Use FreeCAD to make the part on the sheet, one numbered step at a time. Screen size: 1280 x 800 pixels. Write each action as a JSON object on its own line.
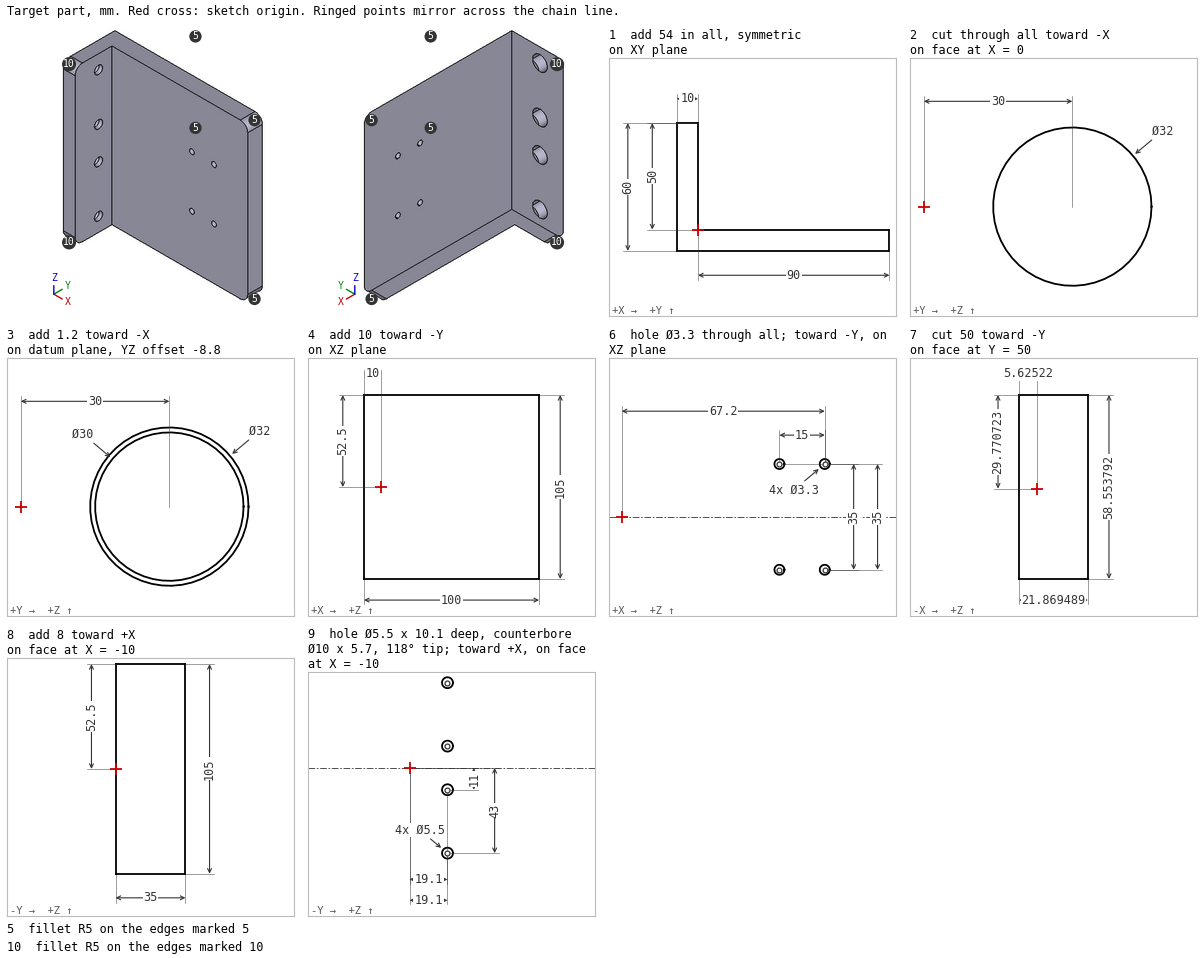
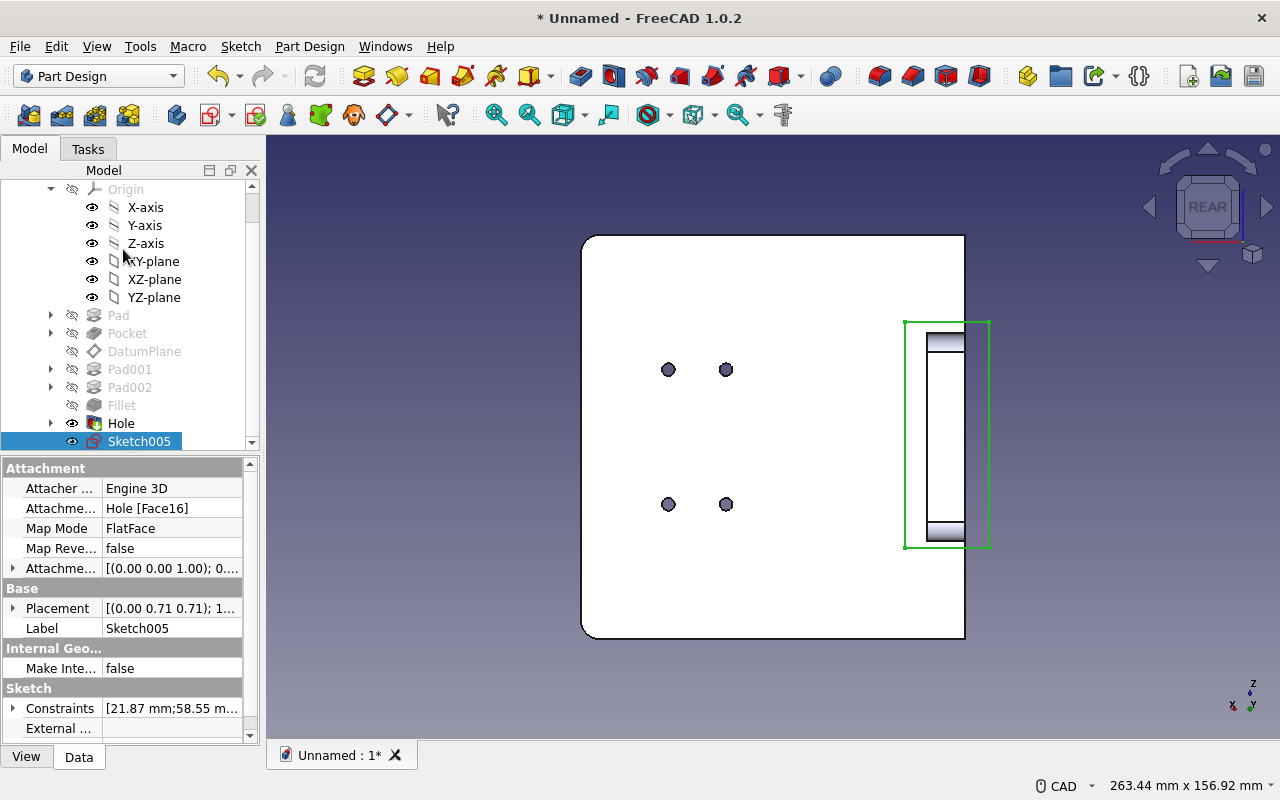
{"action": "left_click", "coordinate": [581, 76]}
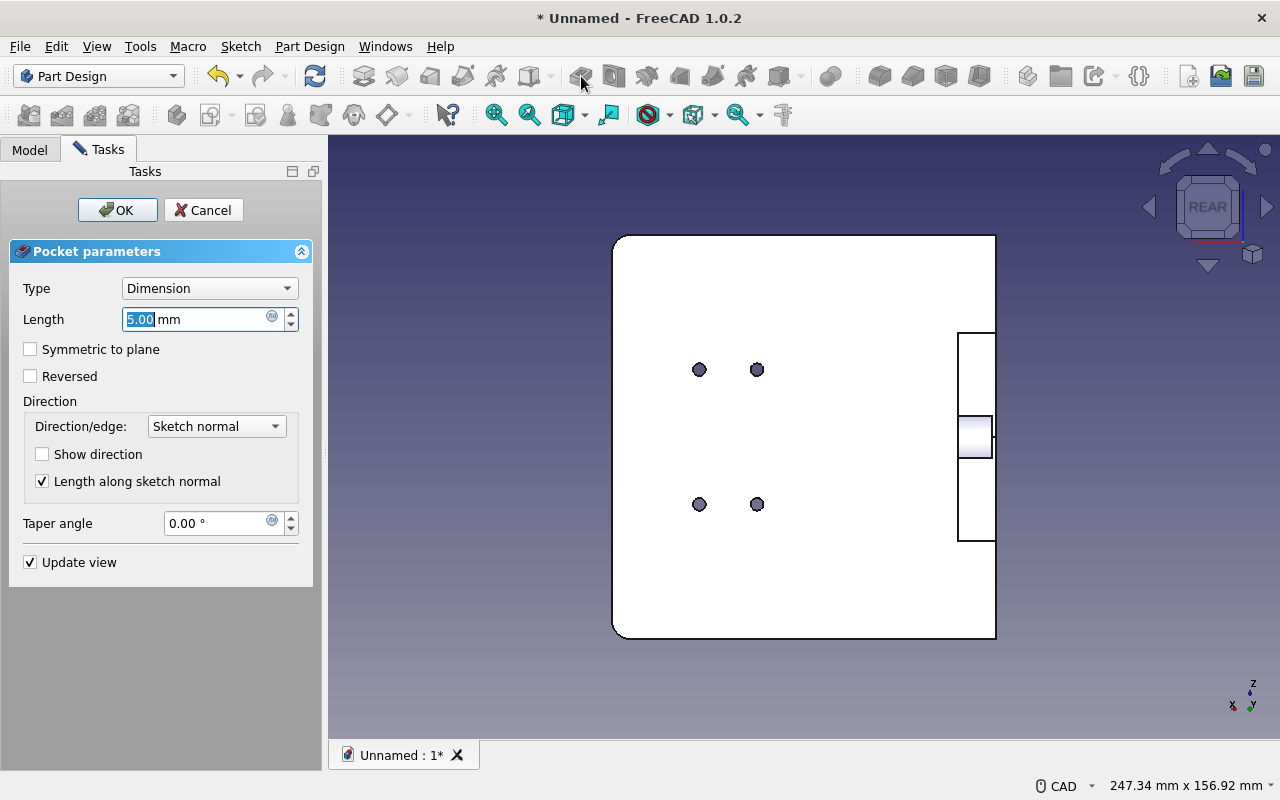
{"action": "type", "text": "50"}
{"action": "key", "text": "Tab"}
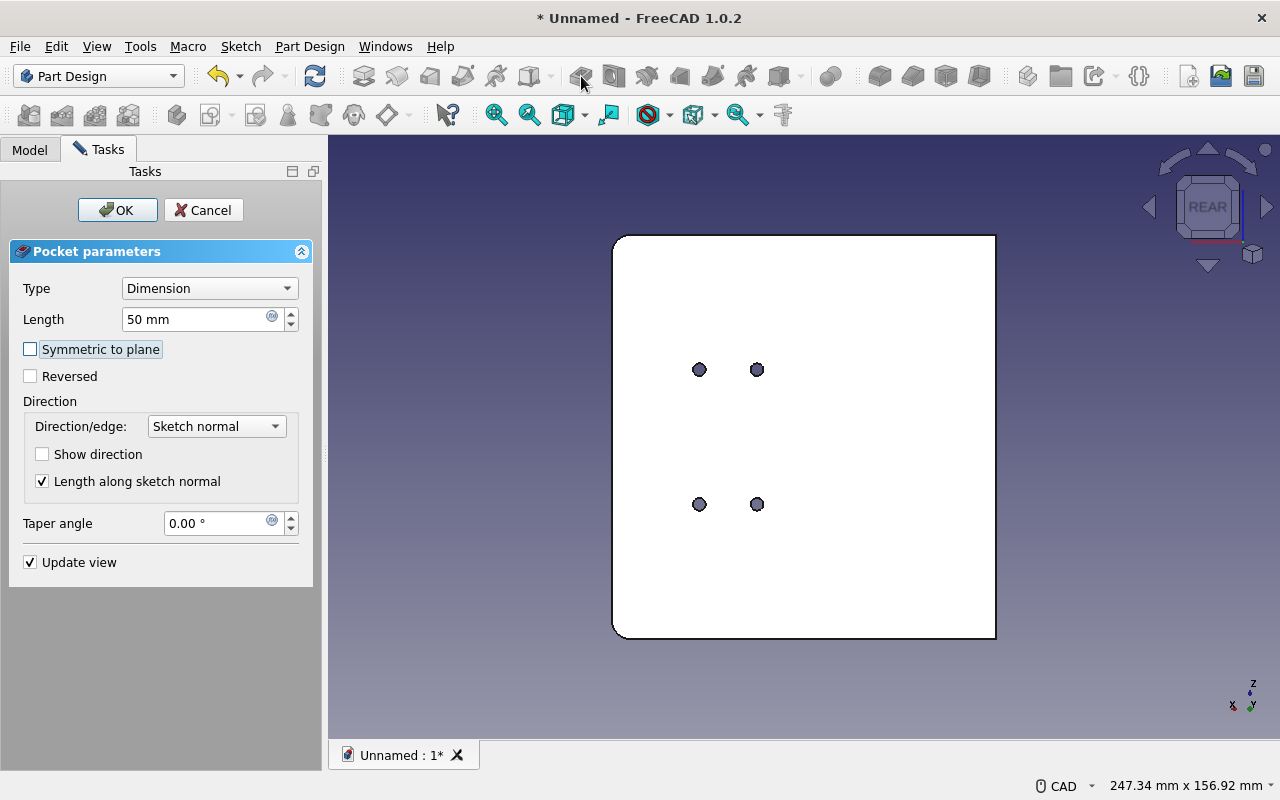
{"action": "left_click", "coordinate": [118, 210]}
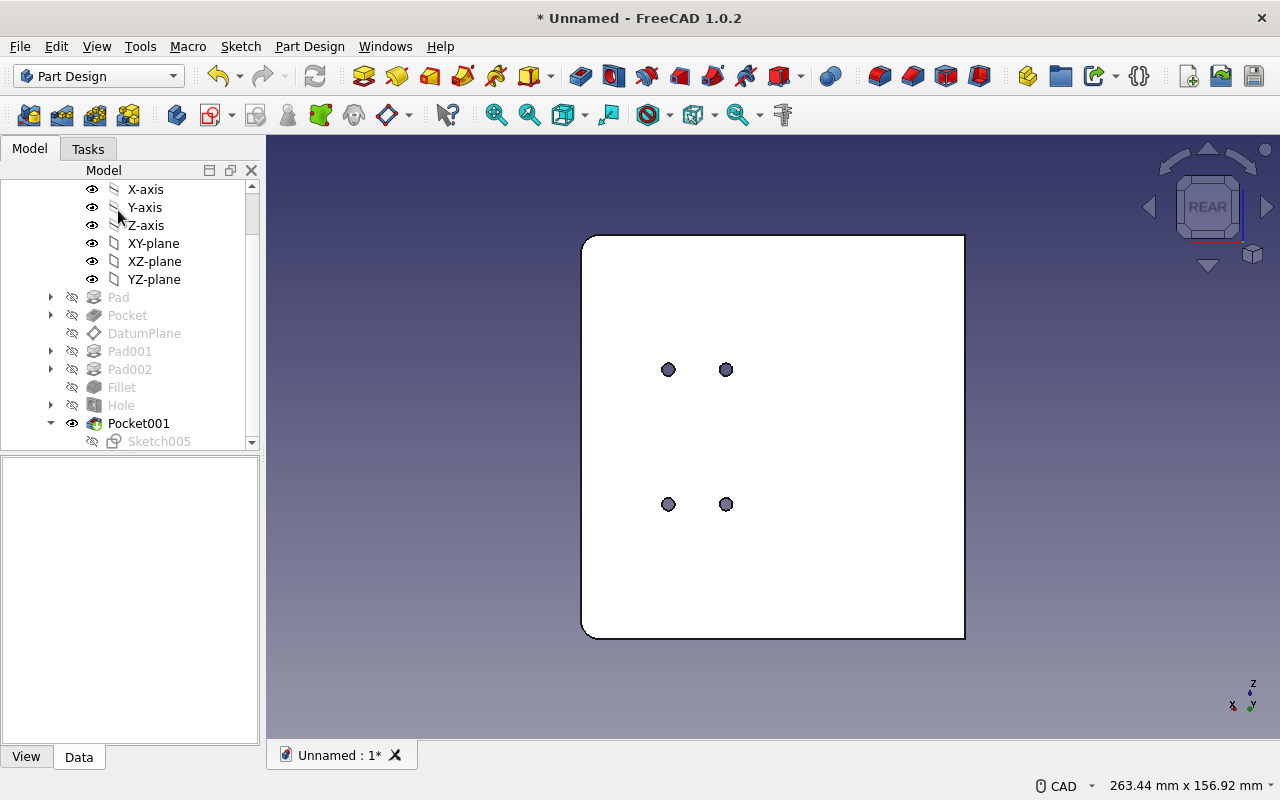
{"action": "key", "text": "6"}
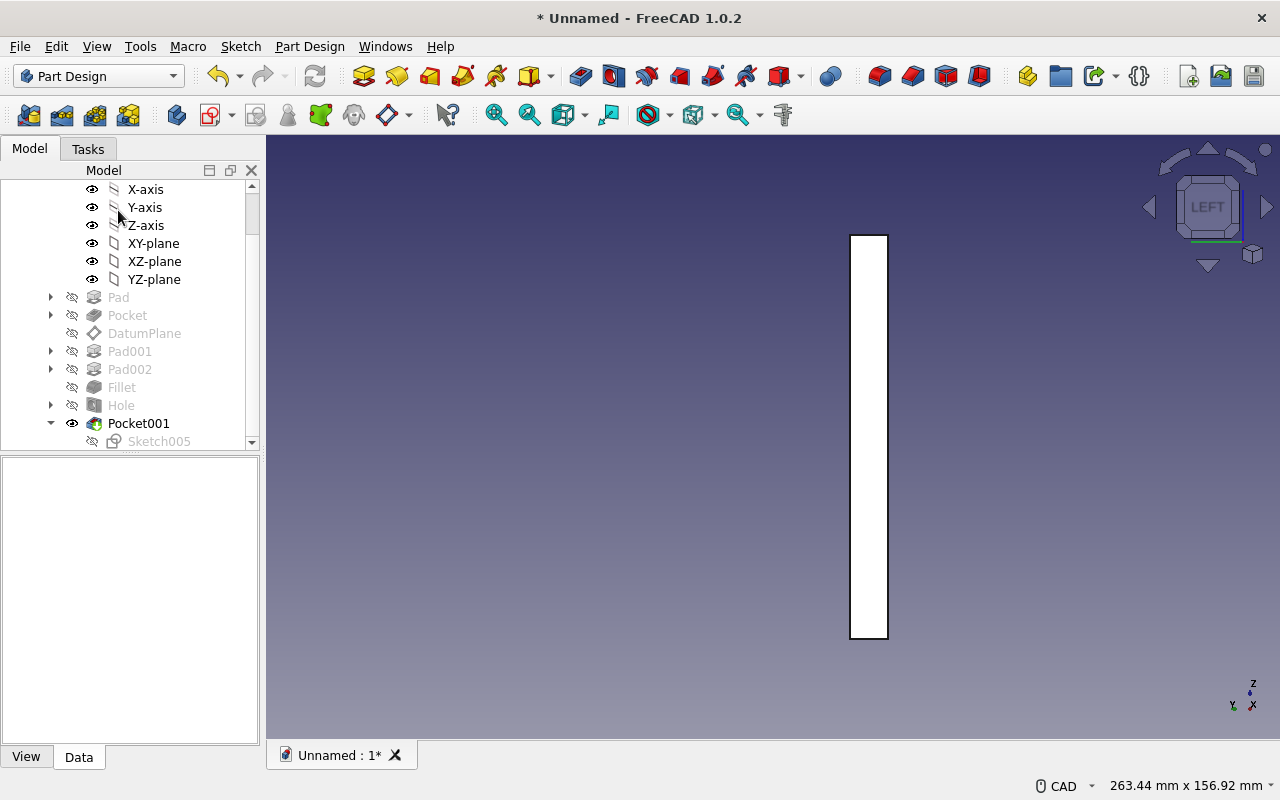
{"action": "left_click", "coordinate": [869, 436]}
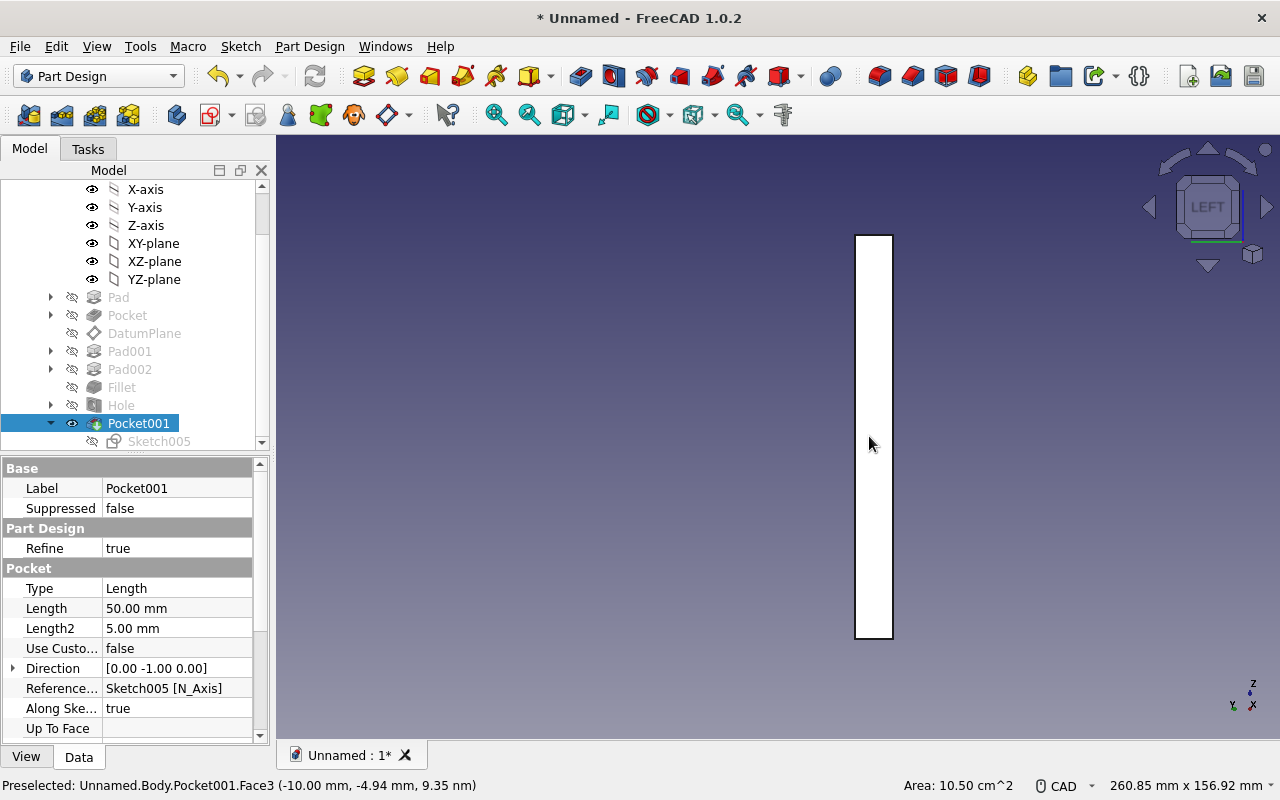
{"action": "left_click", "coordinate": [210, 116]}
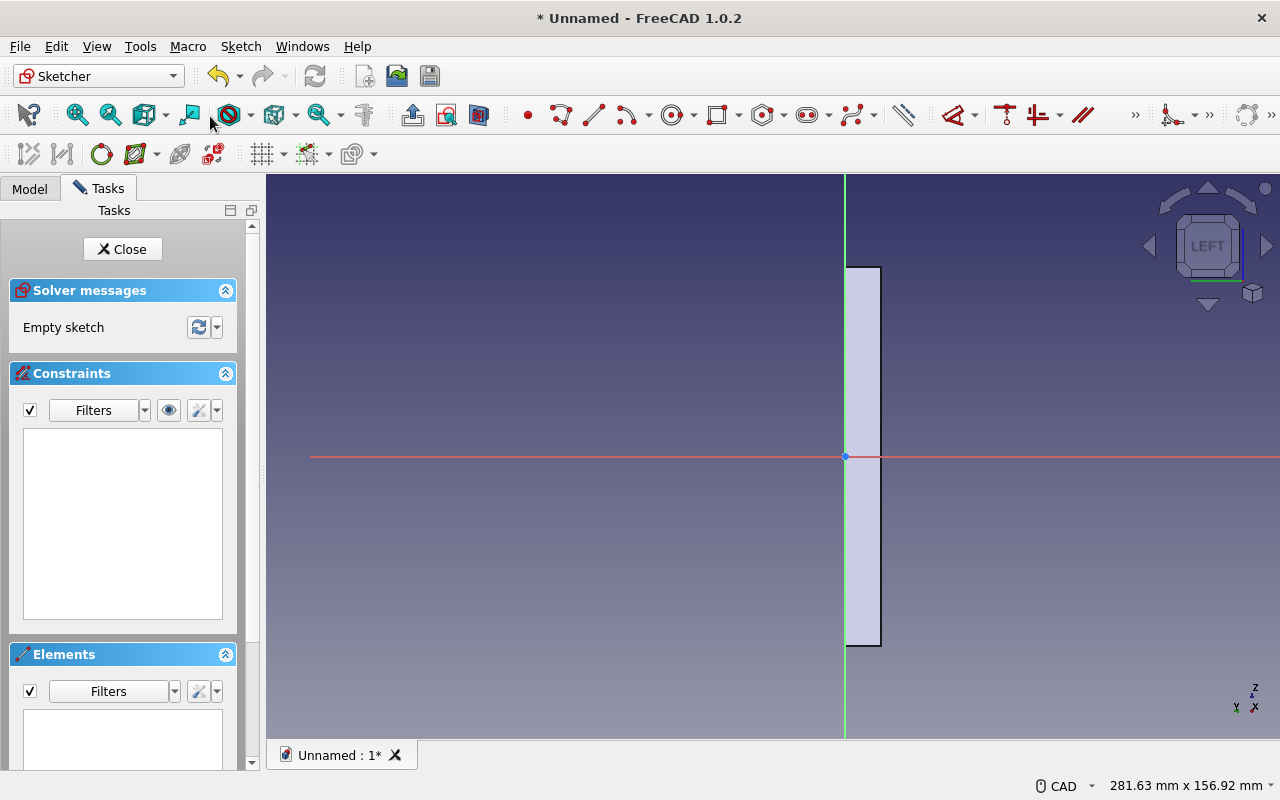
{"action": "left_click", "coordinate": [716, 116]}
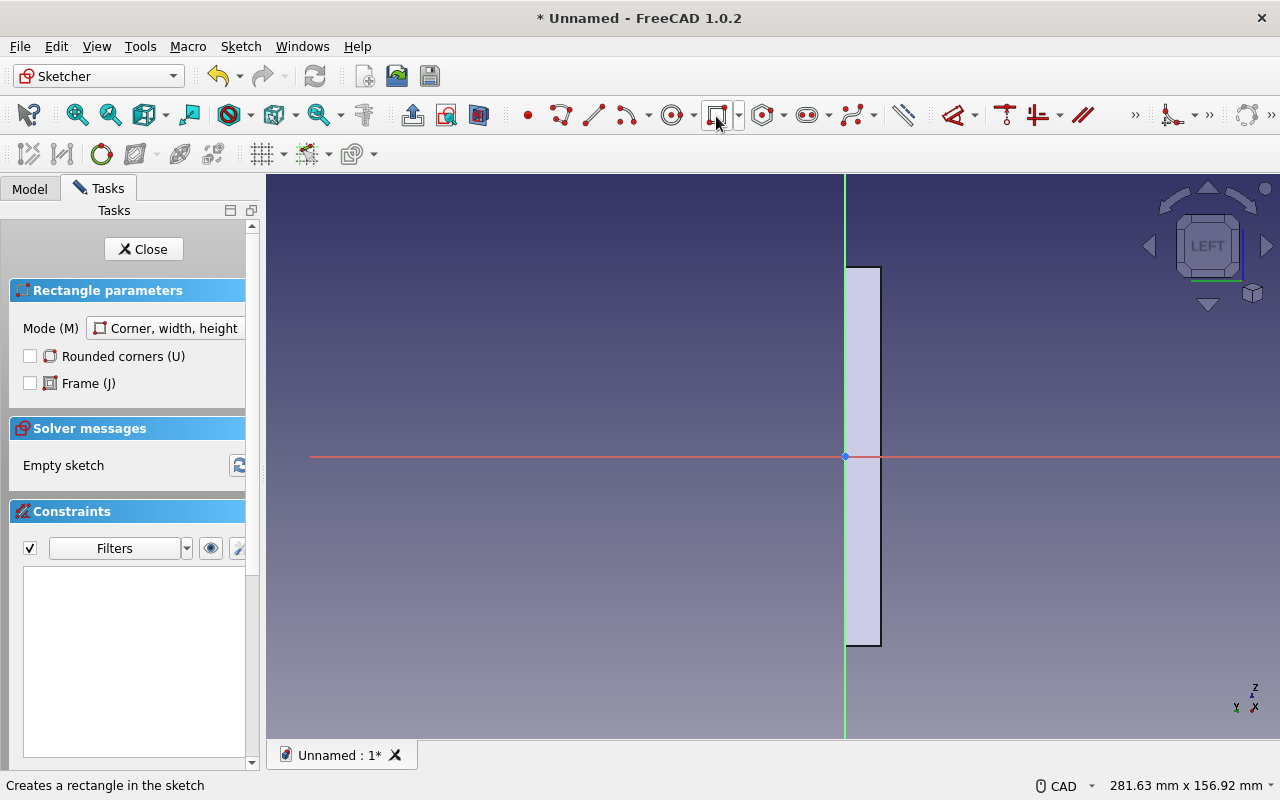
{"action": "left_click", "coordinate": [845, 267]}
{"action": "mouse_move", "coordinate": [971, 646]}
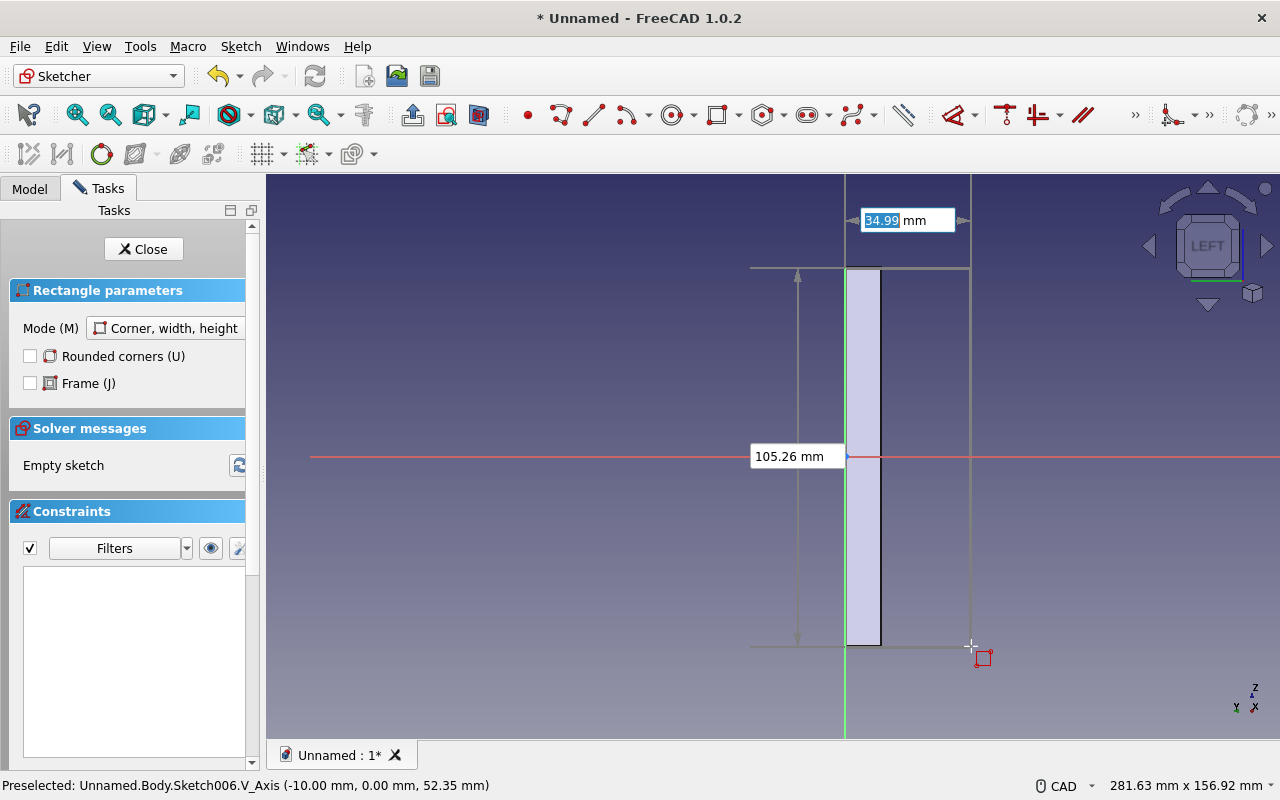
{"action": "type", "text": "35"}
{"action": "key", "text": "Tab"}
{"action": "type", "text": "105"}
{"action": "key", "text": "Return"}
{"action": "key", "text": "Escape"}